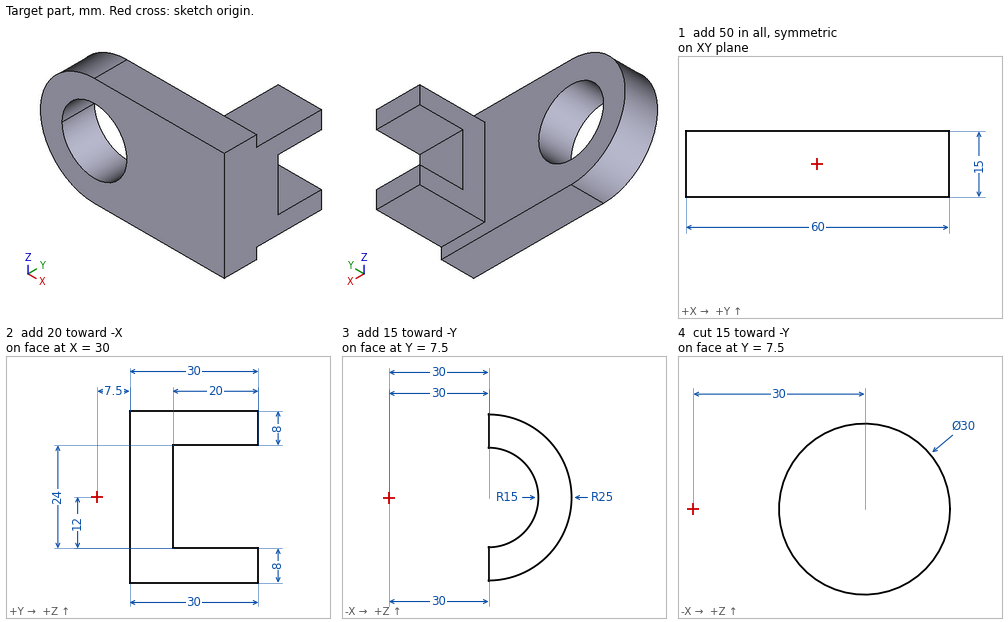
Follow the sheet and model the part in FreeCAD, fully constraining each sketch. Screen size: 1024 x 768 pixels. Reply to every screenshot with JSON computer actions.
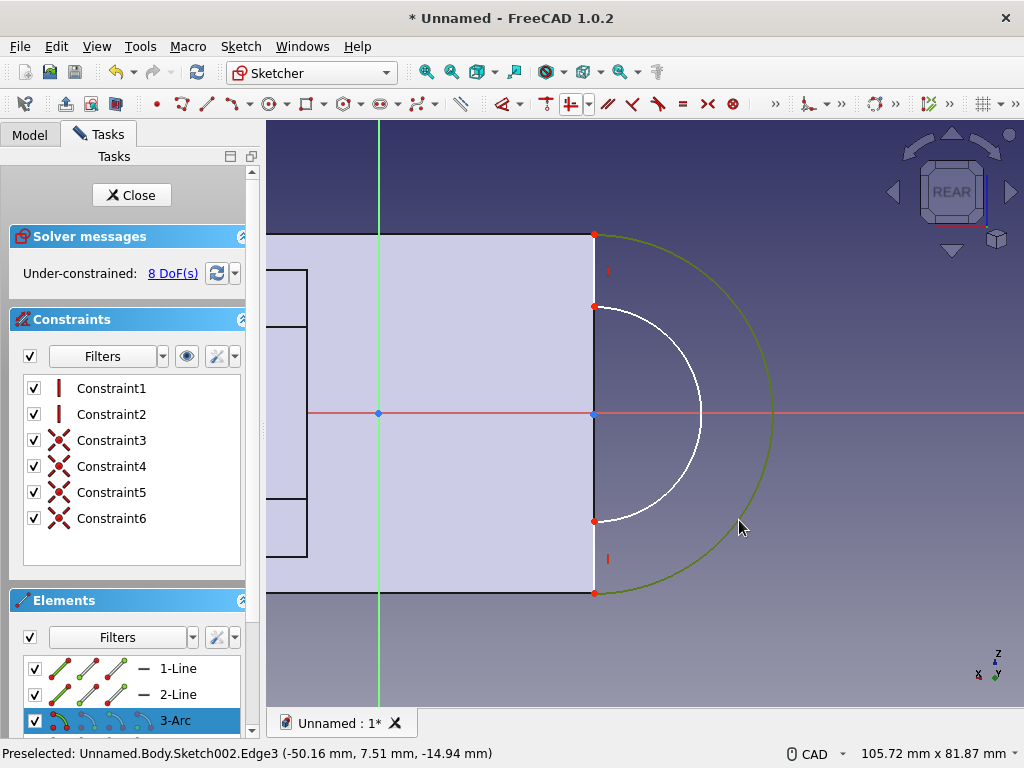
{"action": "left_click", "coordinate": [681, 478]}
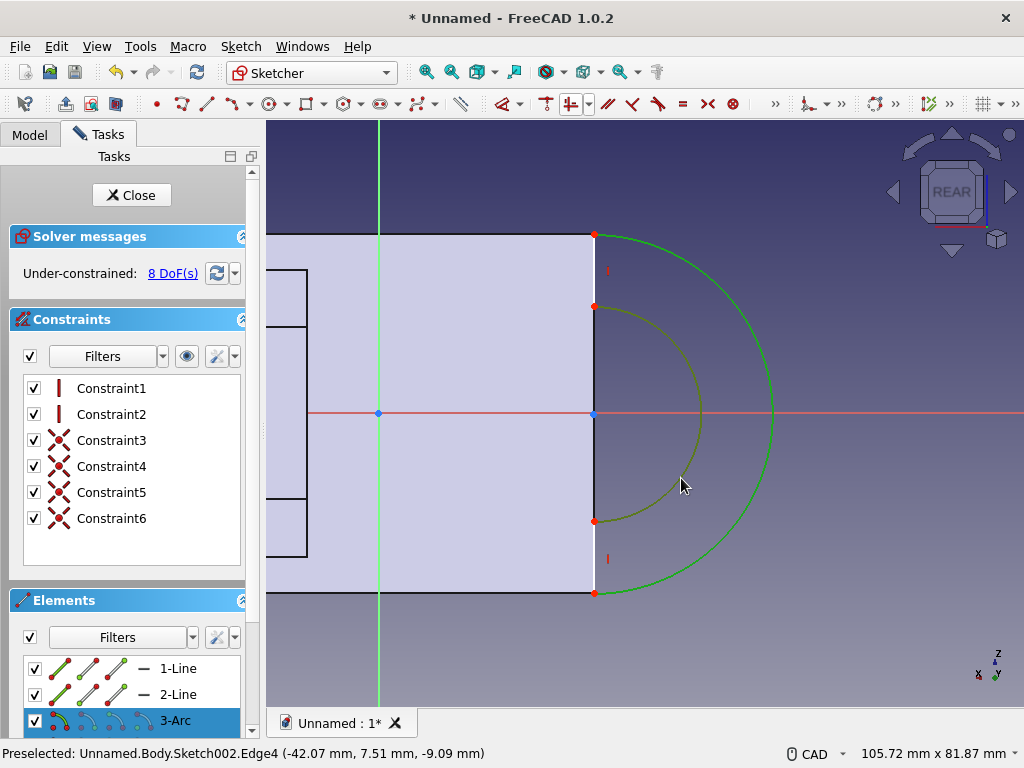
{"action": "key", "text": "c"}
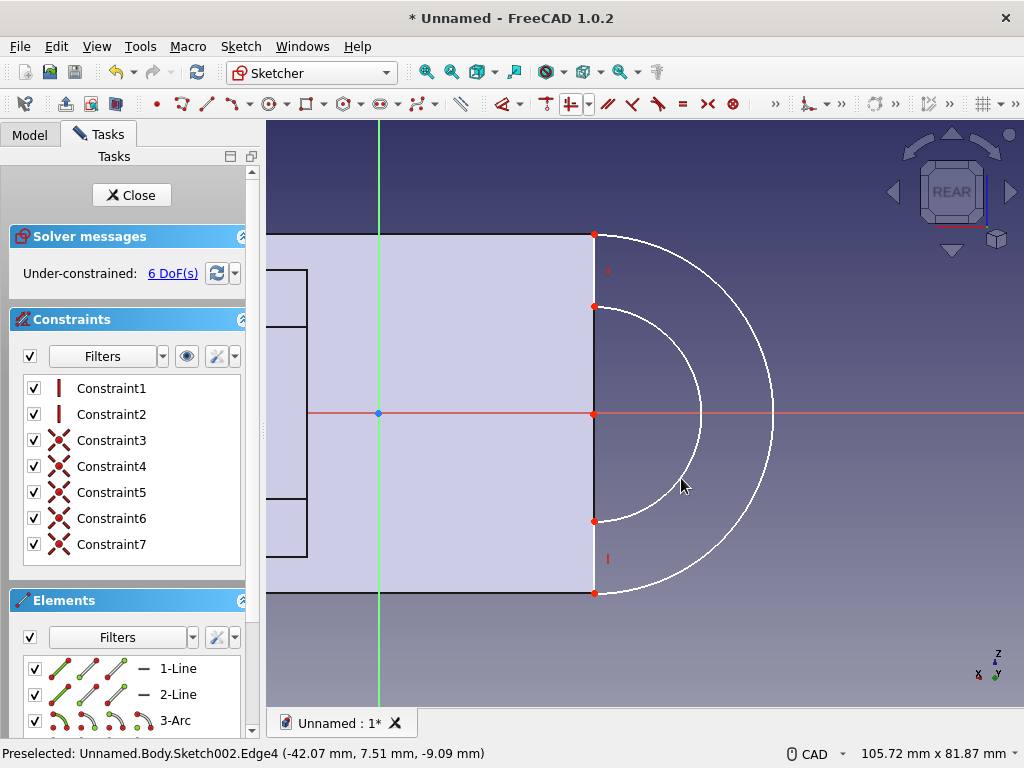
{"action": "left_click", "coordinate": [594, 414]}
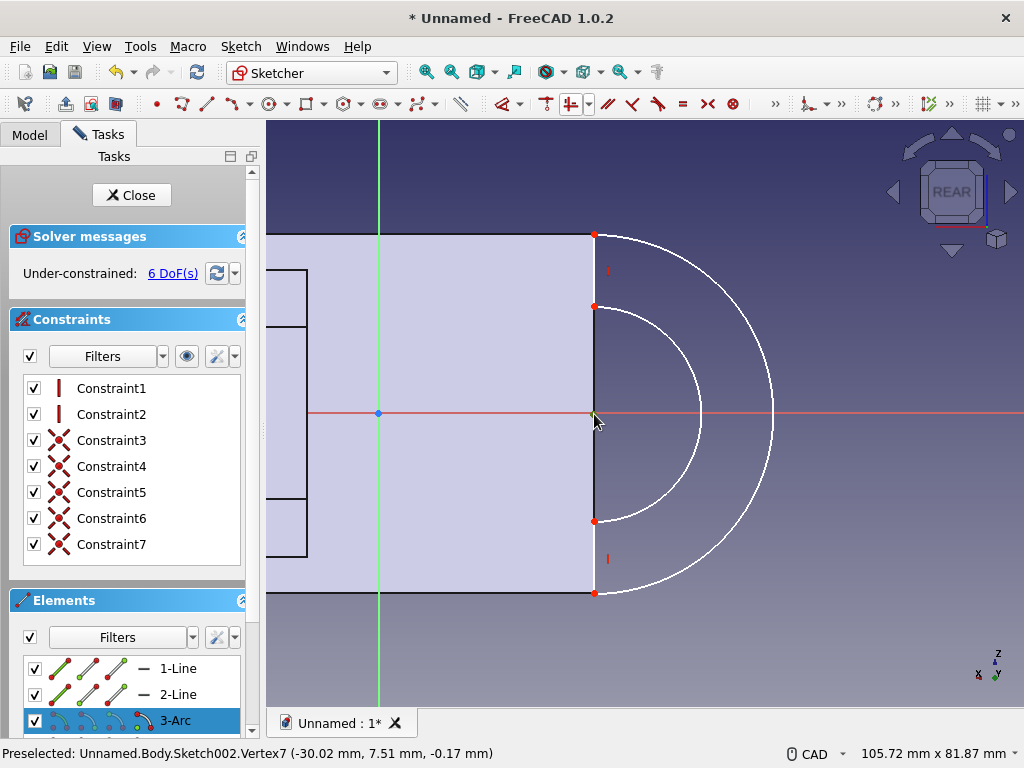
{"action": "left_click", "coordinate": [334, 413]}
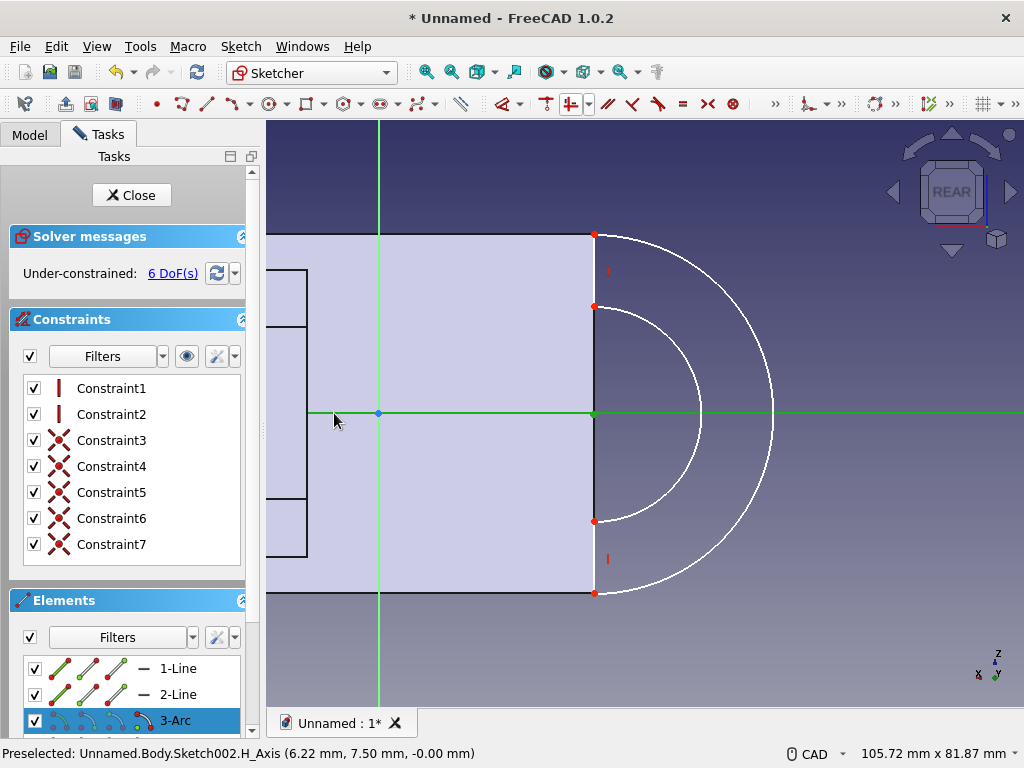
{"action": "key", "text": "c"}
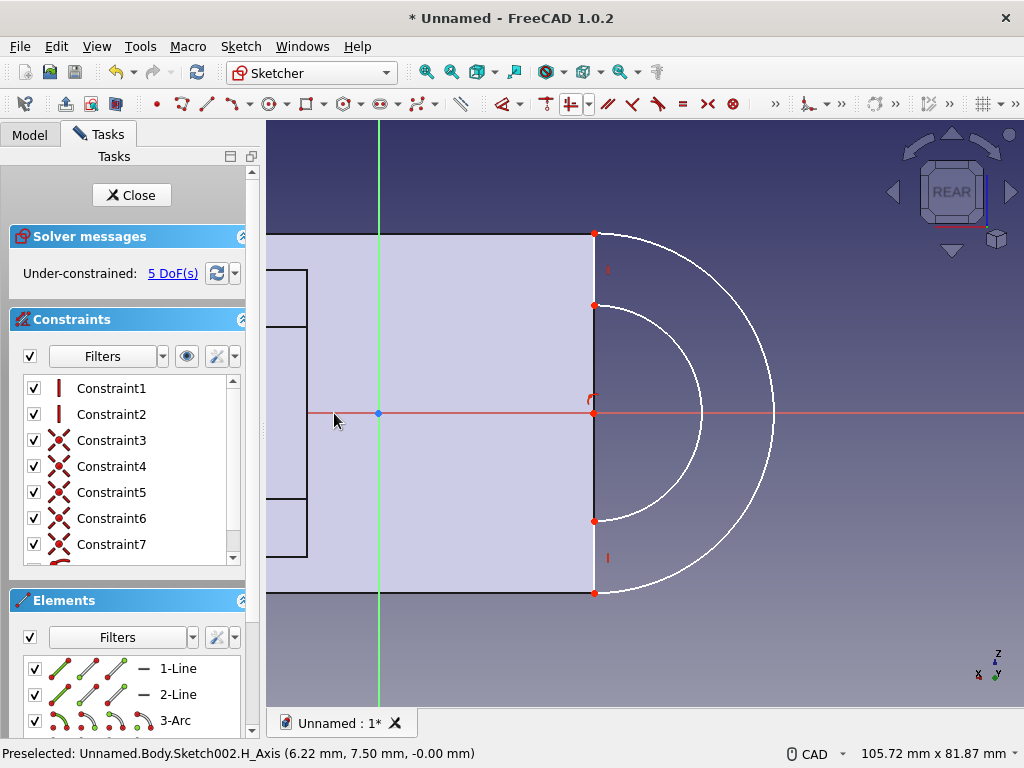
{"action": "key", "text": "d"}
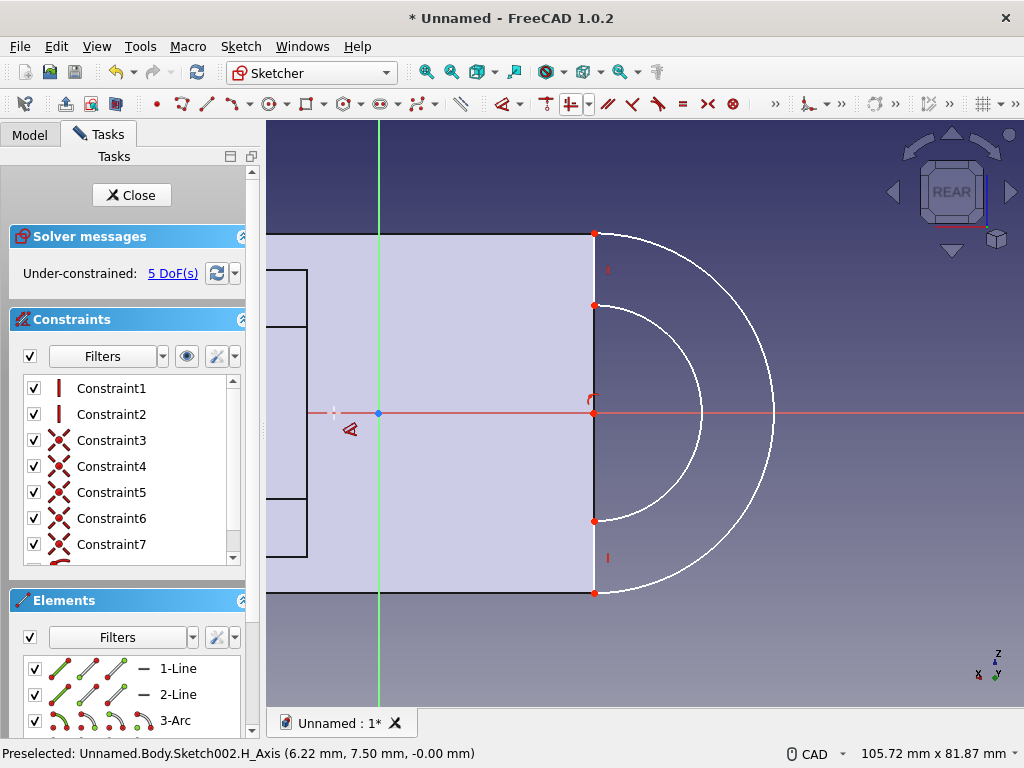
{"action": "left_click", "coordinate": [740, 519]}
{"action": "left_click", "coordinate": [766, 538]}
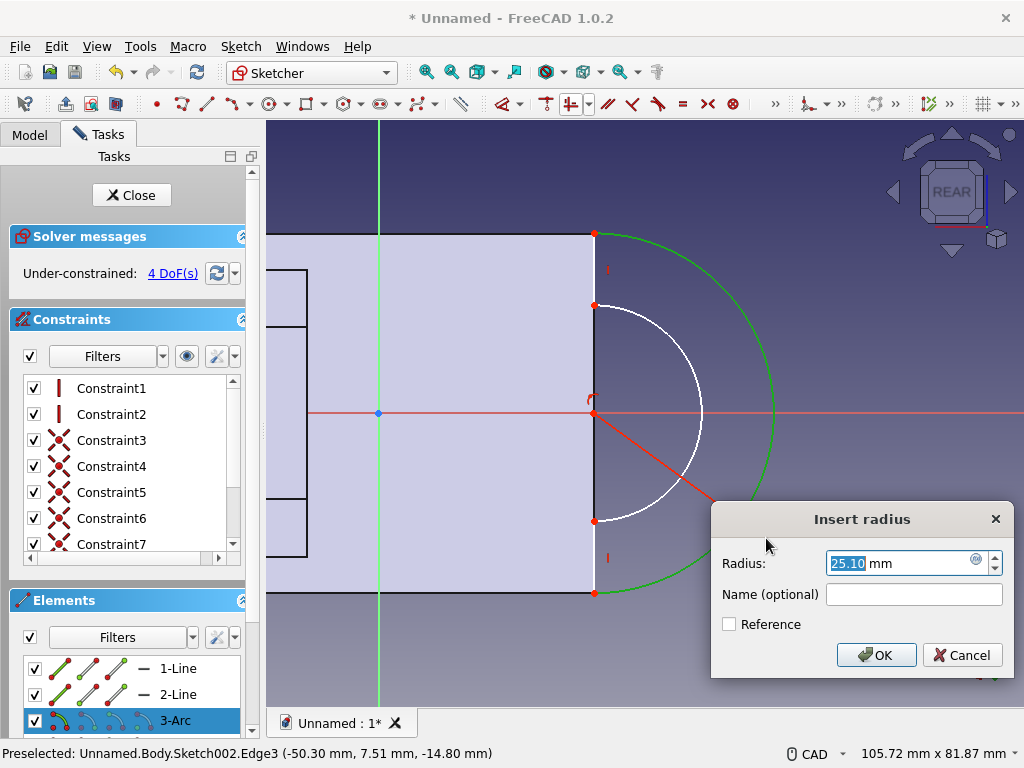
{"action": "type", "text": "25"}
{"action": "key", "text": "Return"}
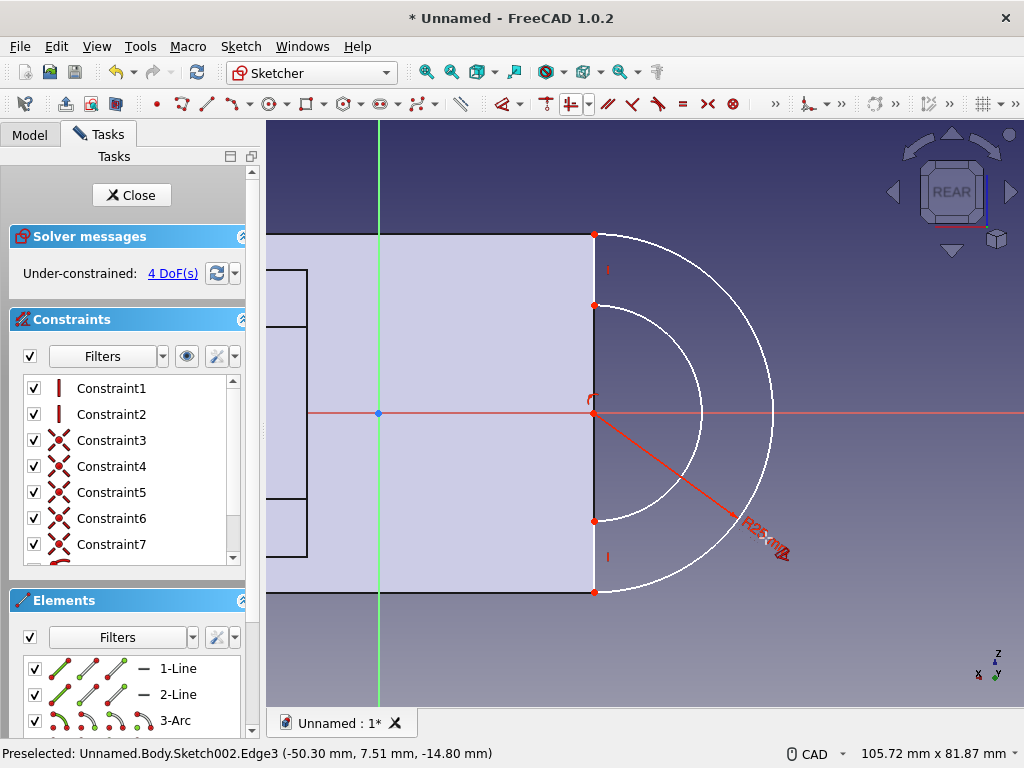
{"action": "left_click", "coordinate": [681, 477]}
{"action": "left_click", "coordinate": [707, 496]}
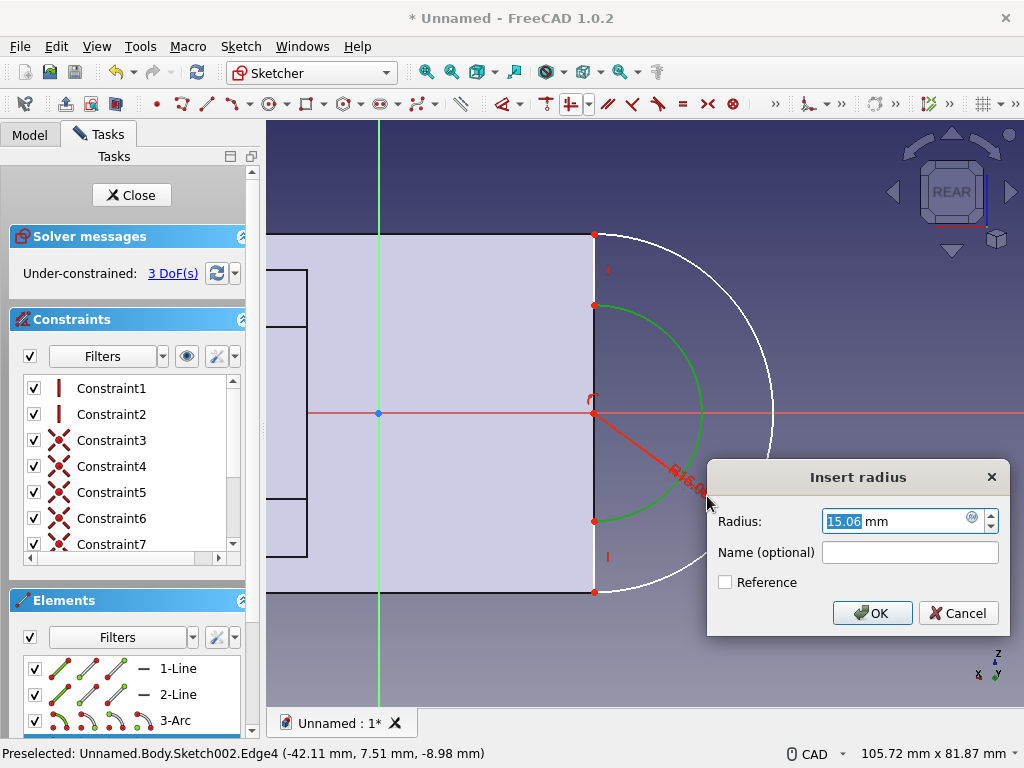
{"action": "type", "text": "15"}
{"action": "key", "text": "Return"}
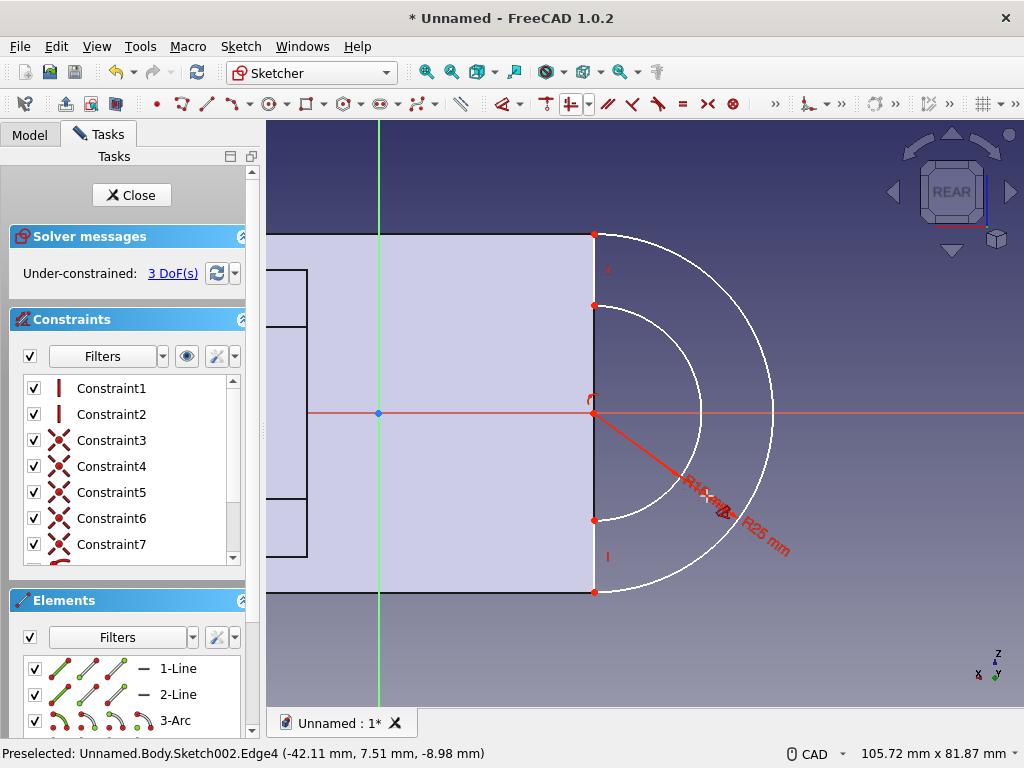
{"action": "left_click", "coordinate": [594, 521]}
{"action": "left_click", "coordinate": [486, 555]}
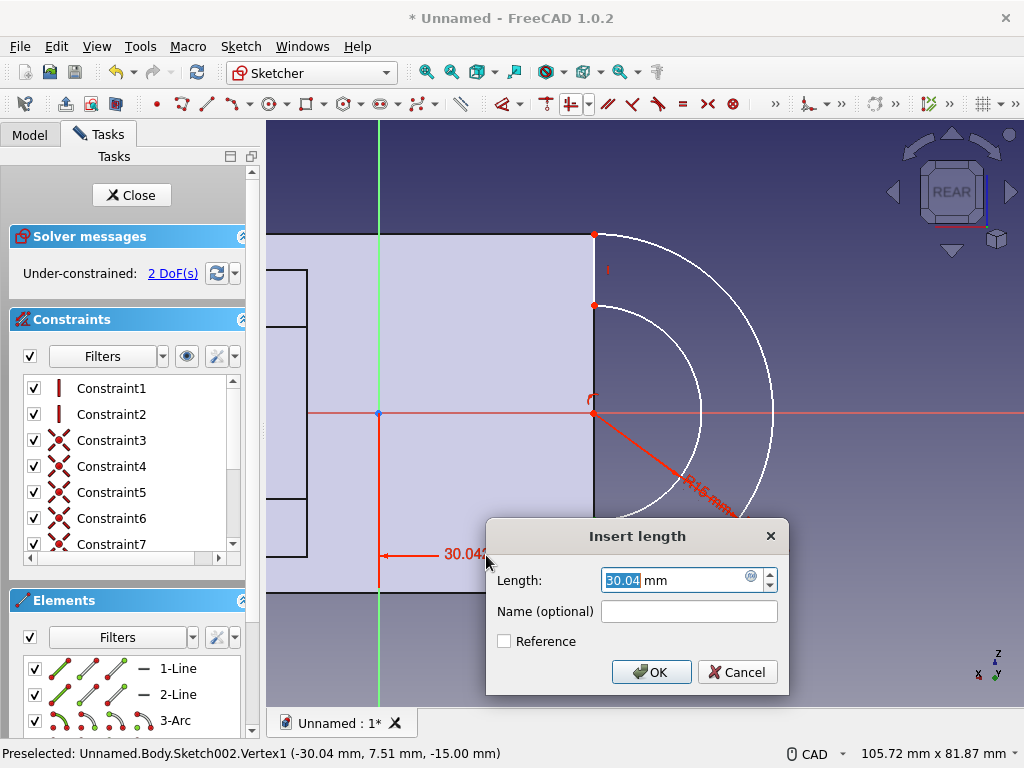
{"action": "type", "text": "30"}
{"action": "key", "text": "Return"}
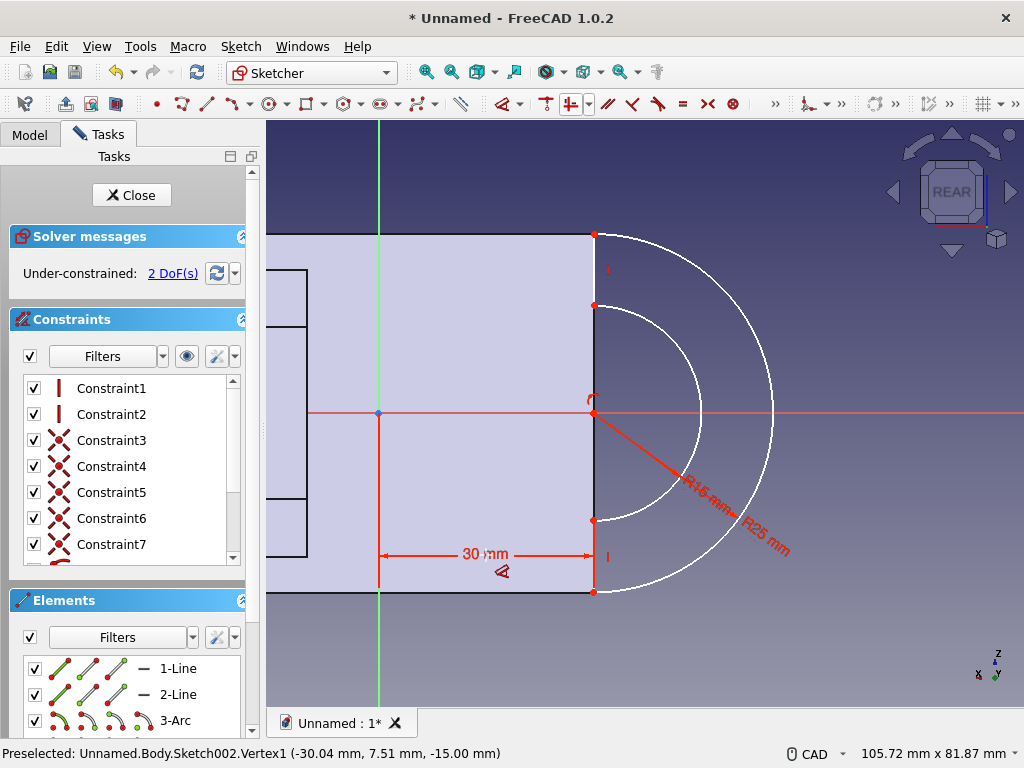
{"action": "left_click", "coordinate": [594, 234]}
{"action": "left_click", "coordinate": [486, 200]}